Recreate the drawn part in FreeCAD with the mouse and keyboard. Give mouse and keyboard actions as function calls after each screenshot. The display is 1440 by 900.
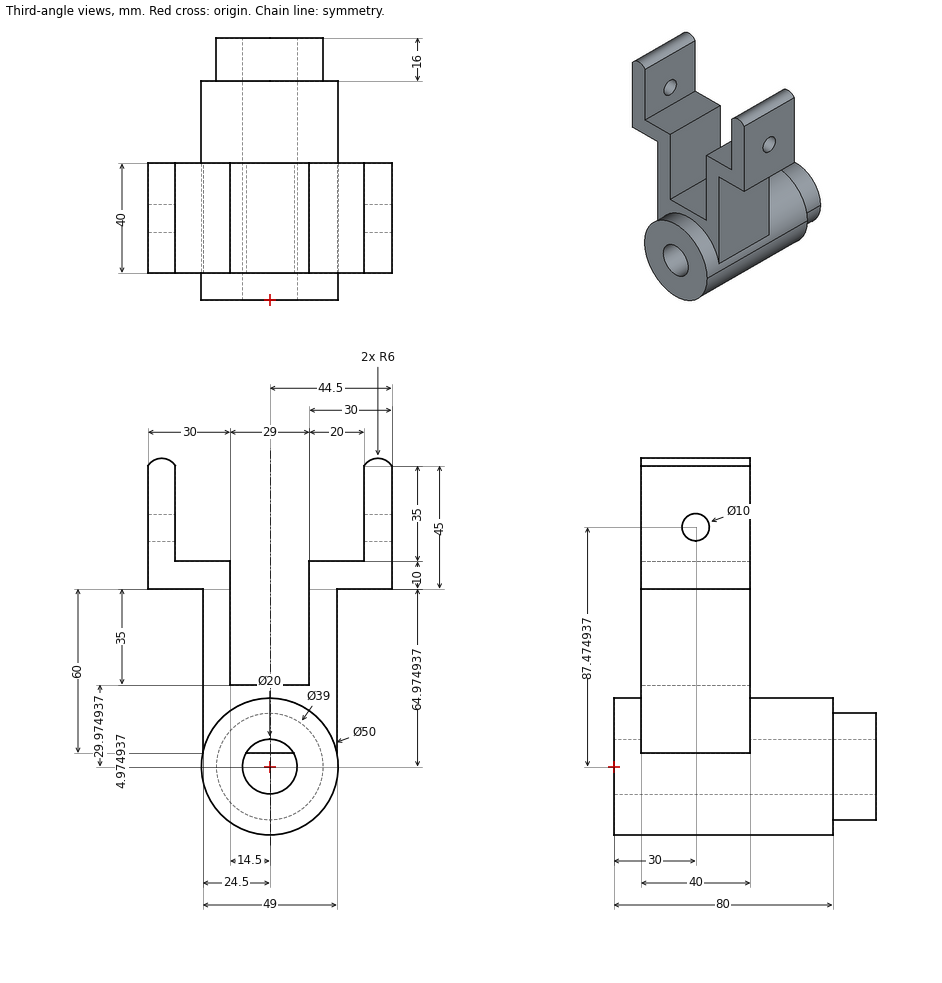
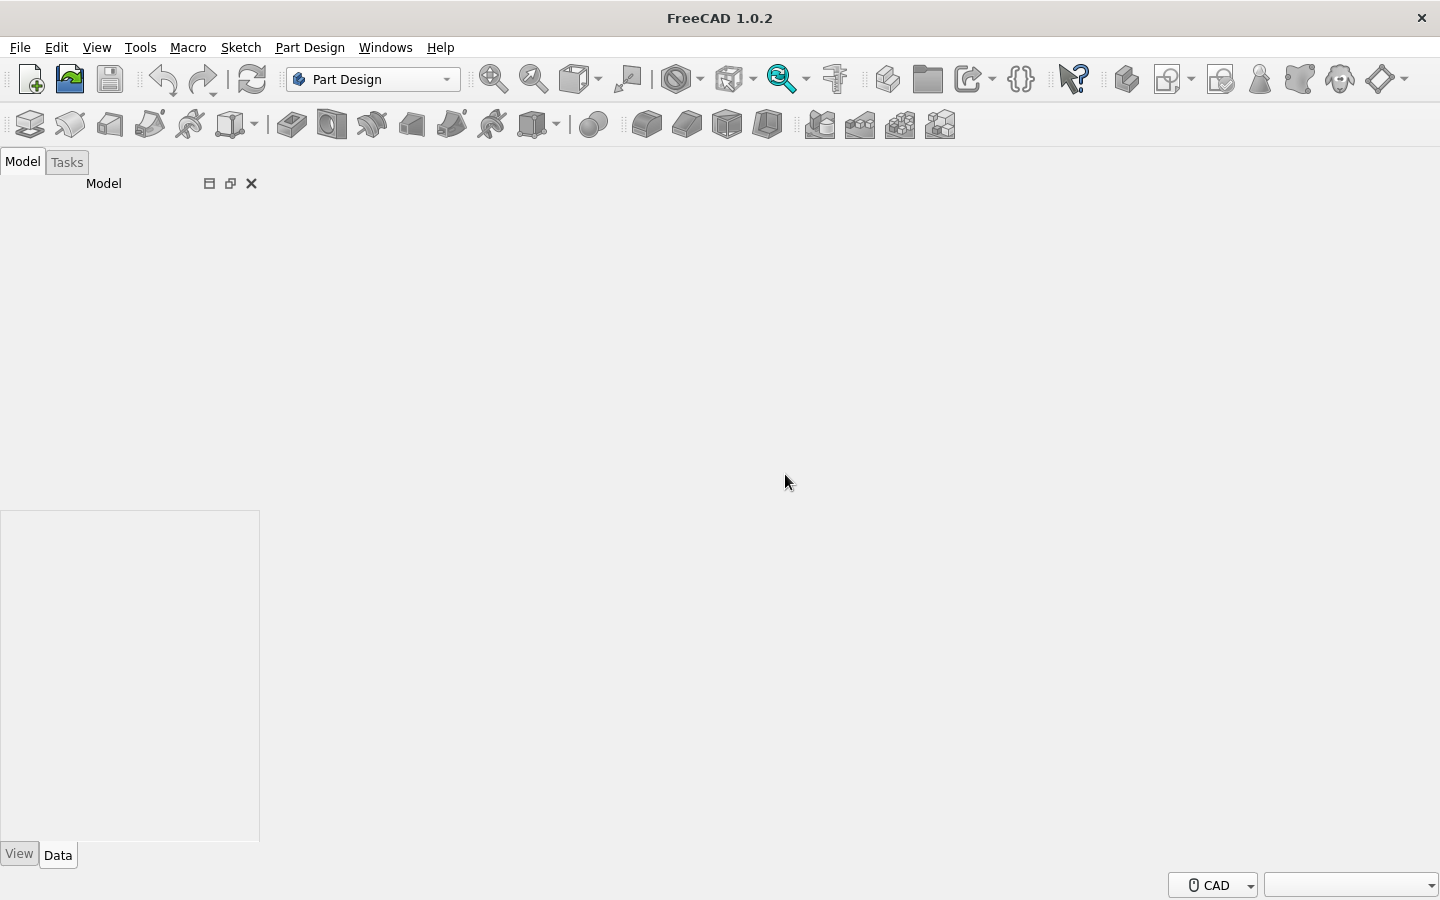
click(30, 80)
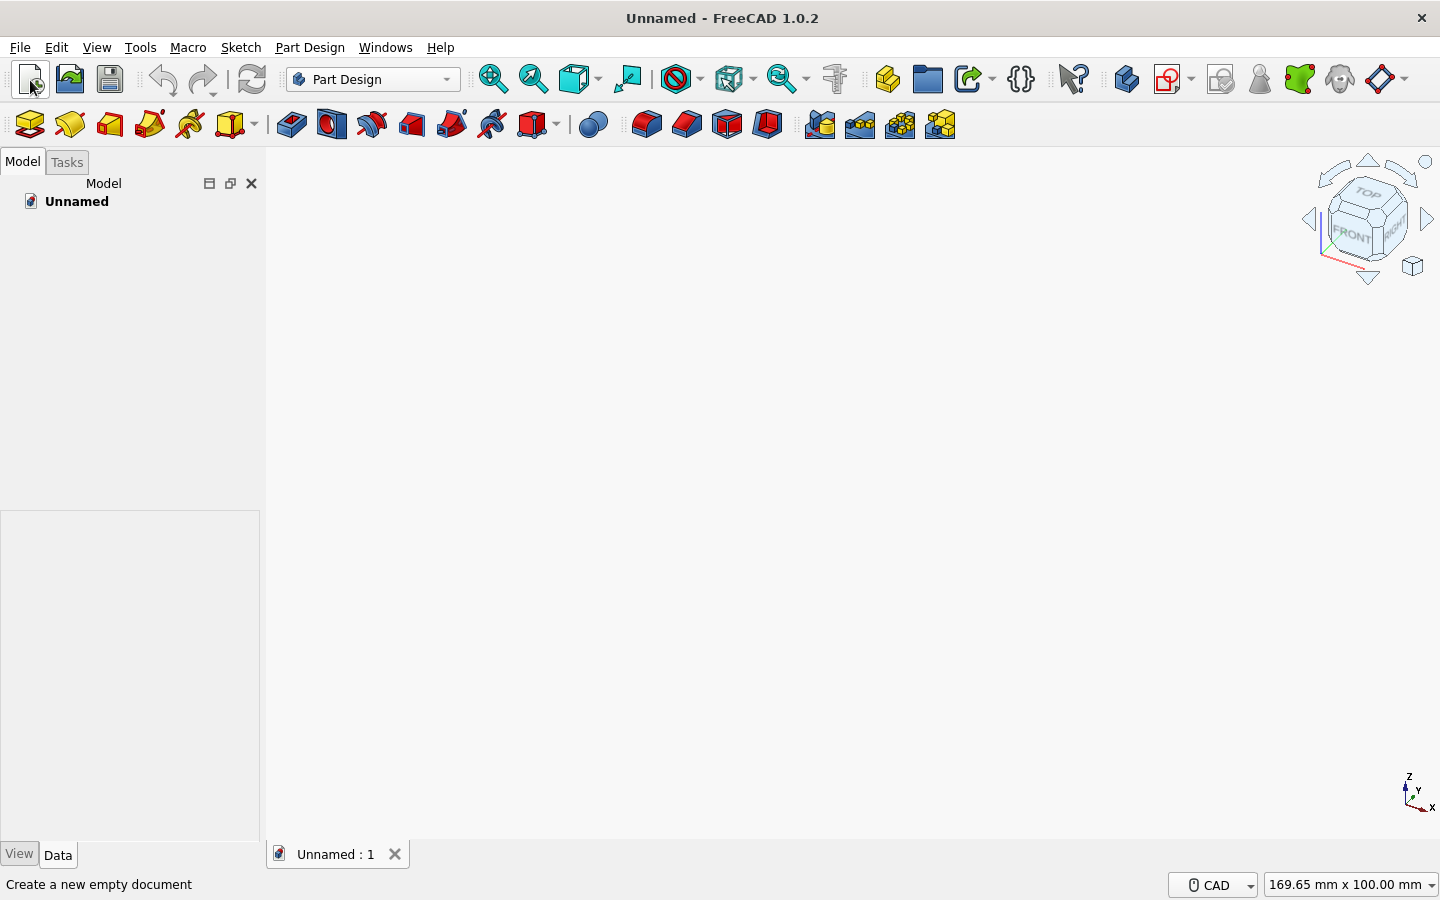
click(1168, 80)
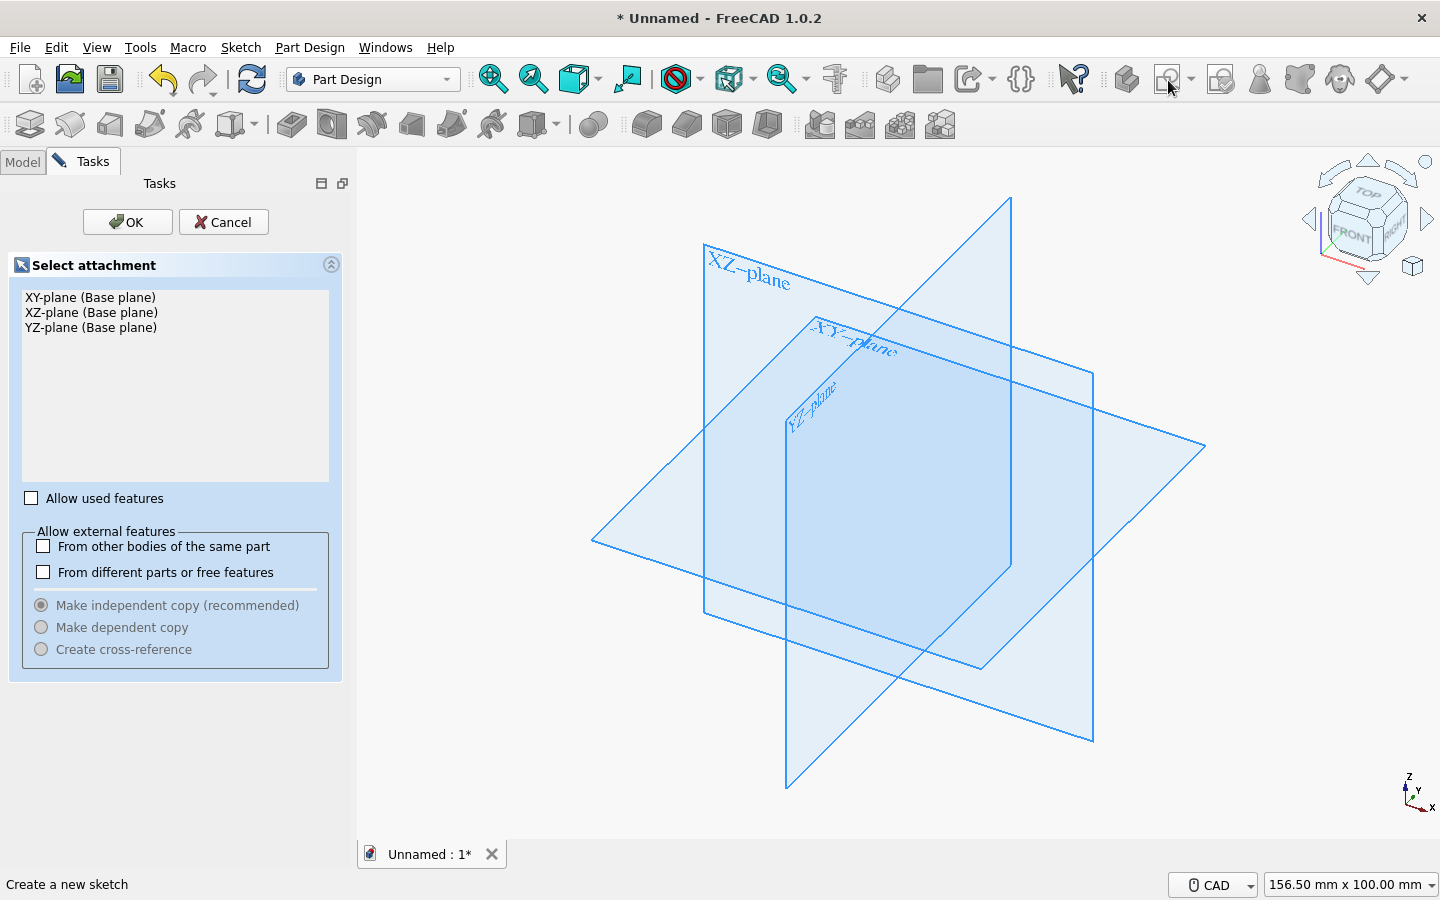
click(82, 312)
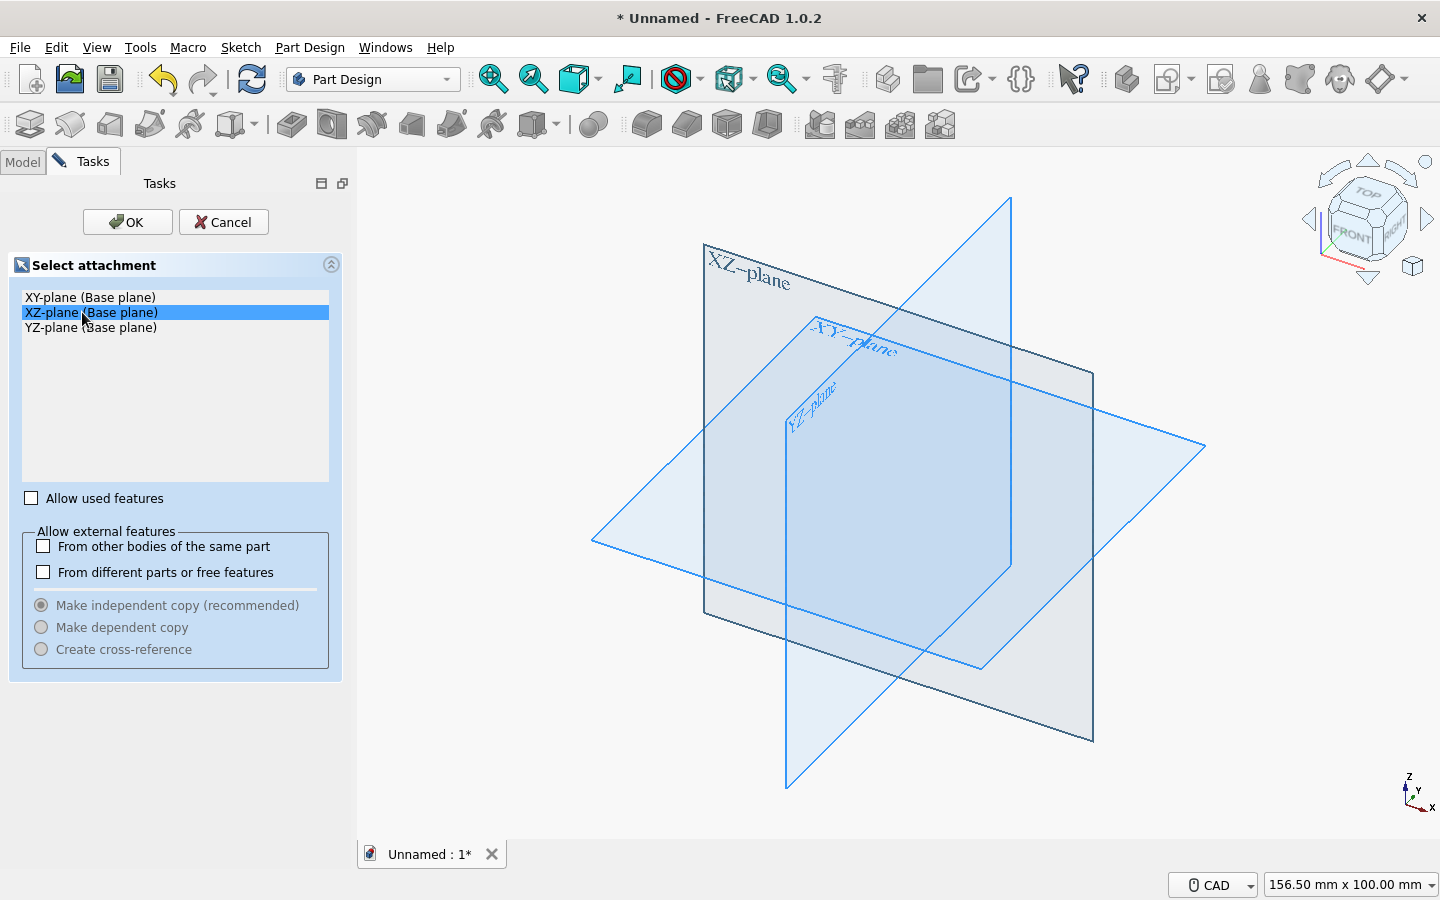
click(128, 222)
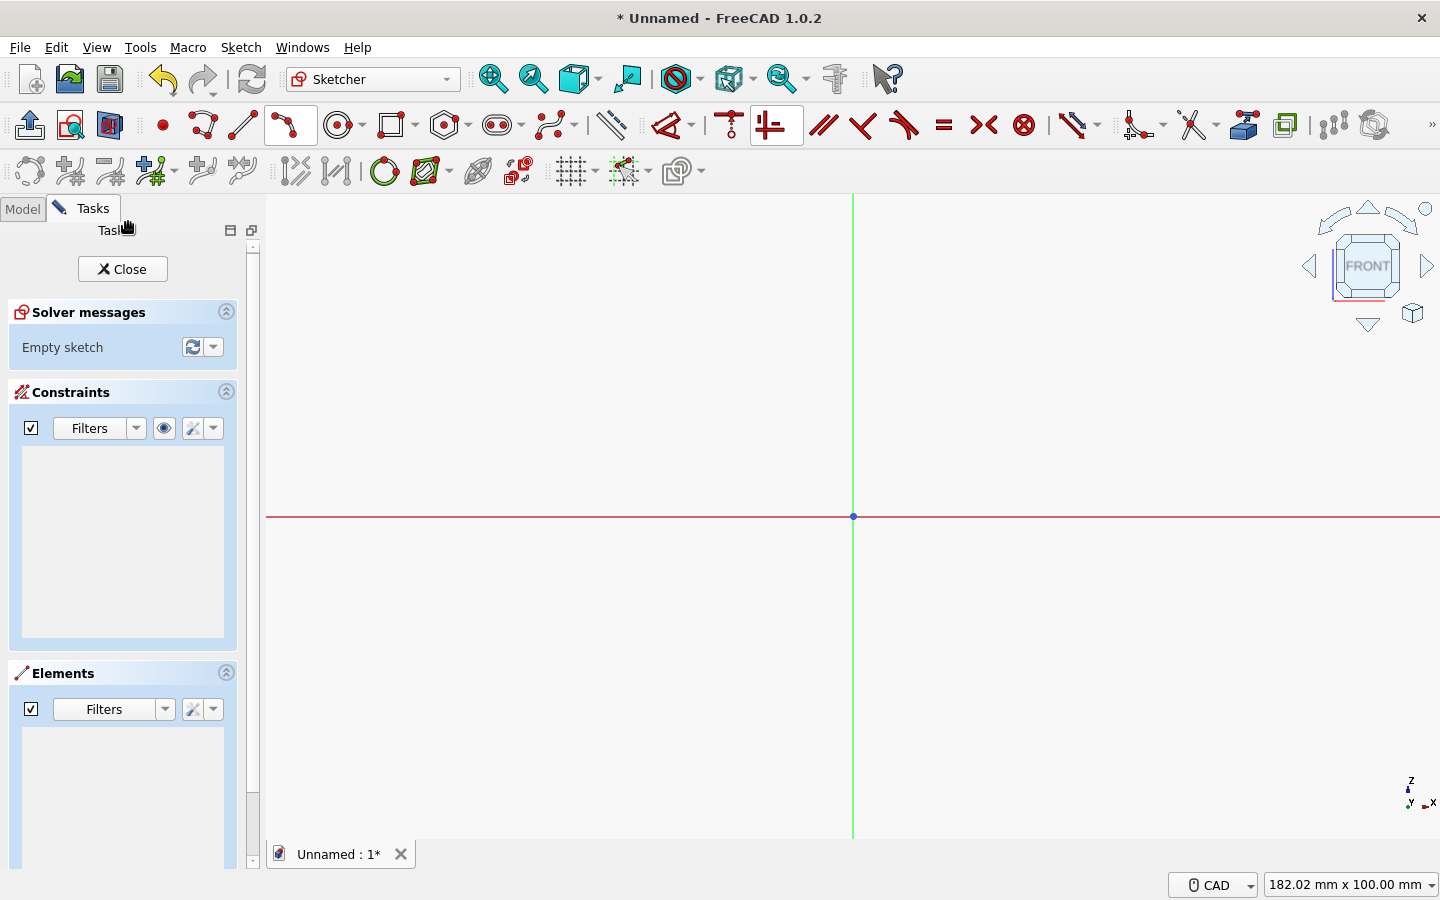
click(338, 126)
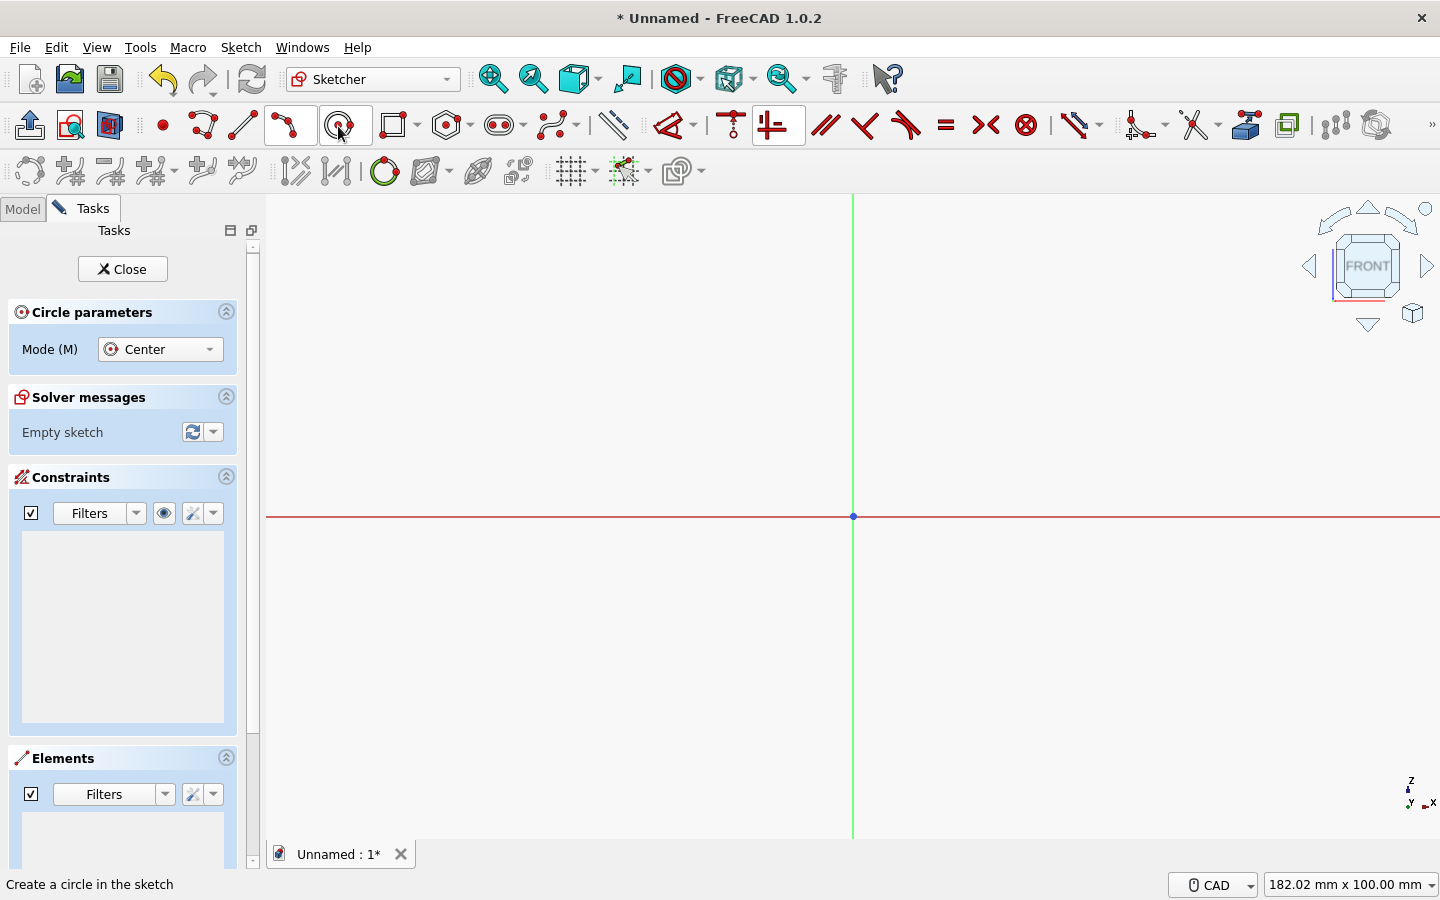
click(853, 516)
click(967, 402)
key(Escape)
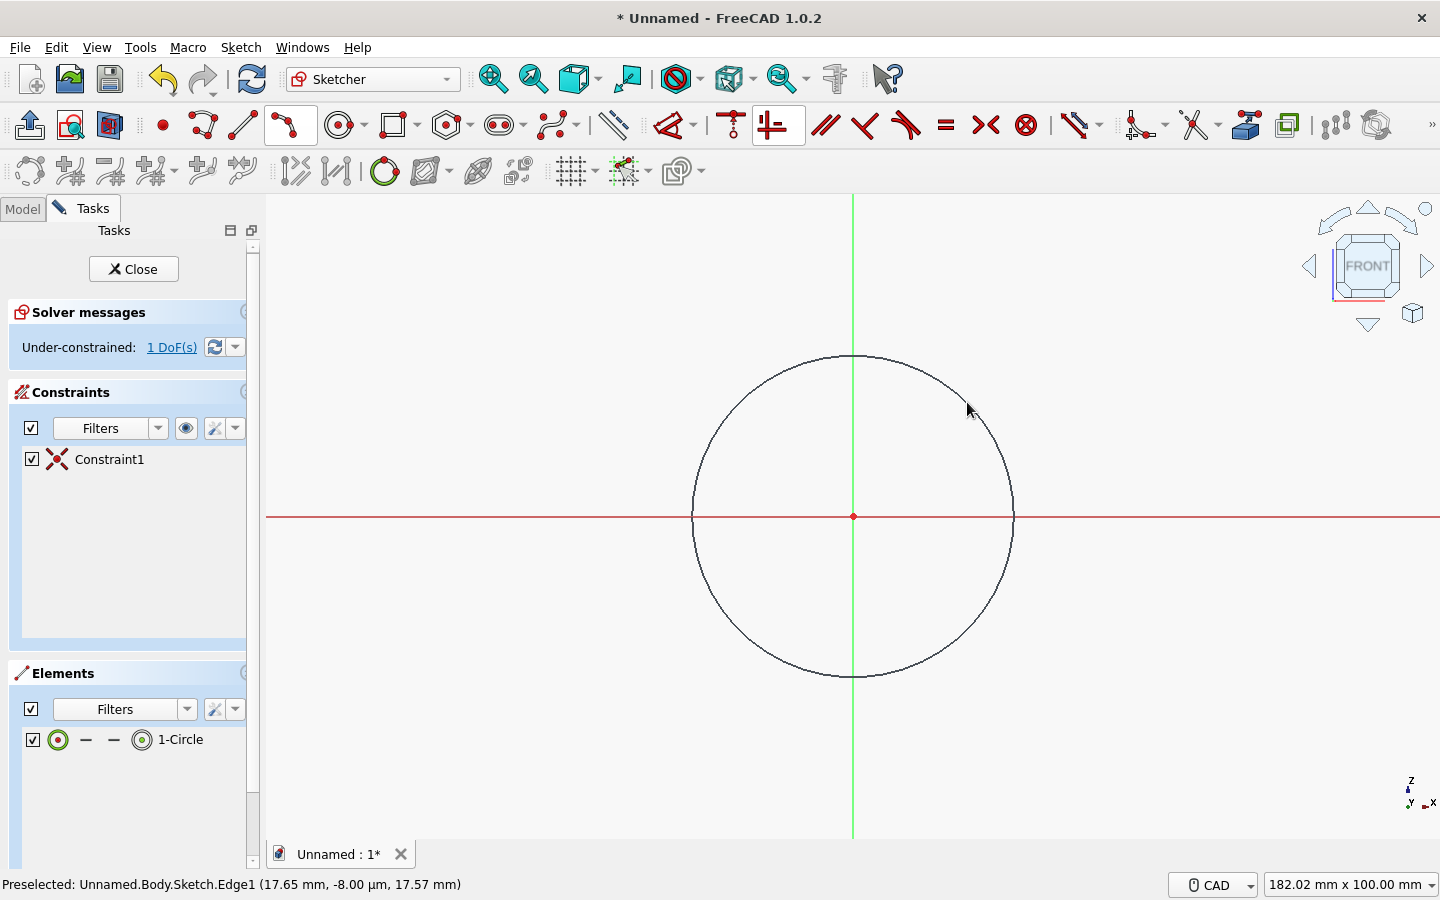
click(668, 126)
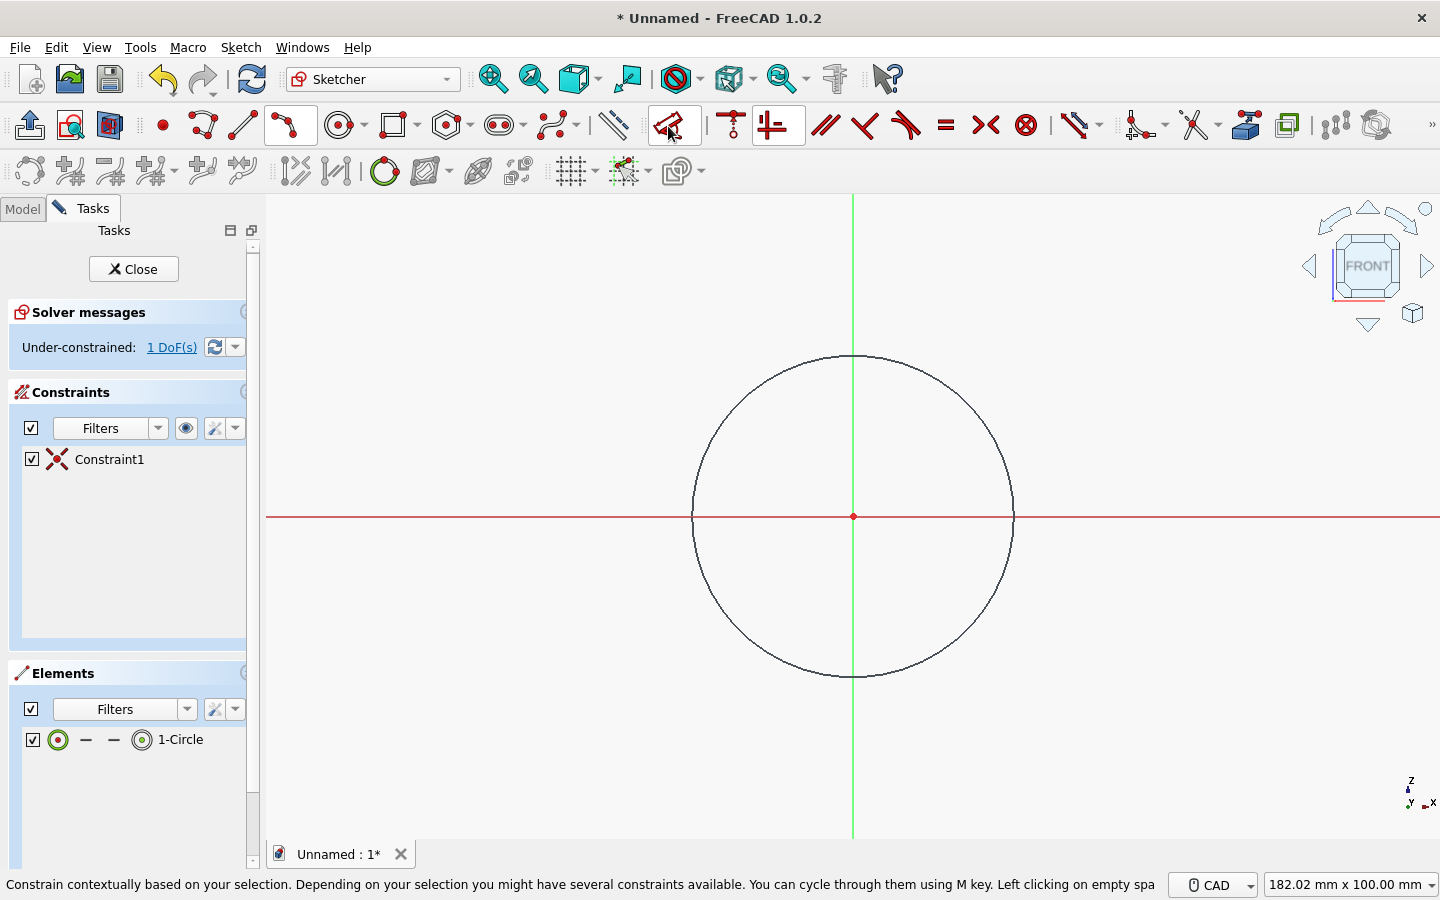
click(966, 402)
click(988, 379)